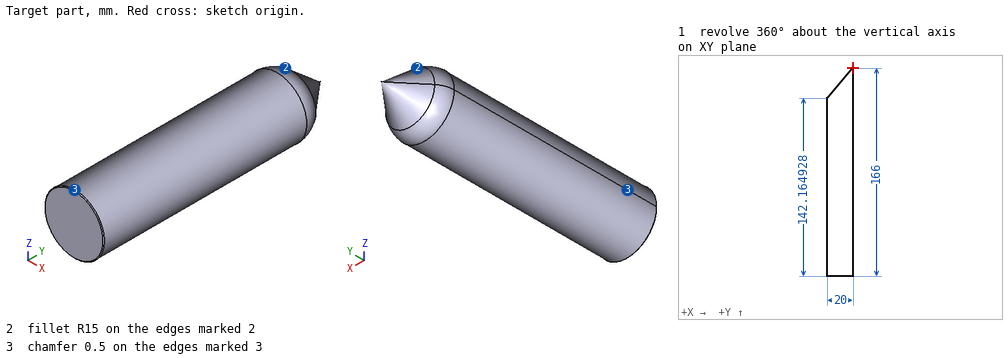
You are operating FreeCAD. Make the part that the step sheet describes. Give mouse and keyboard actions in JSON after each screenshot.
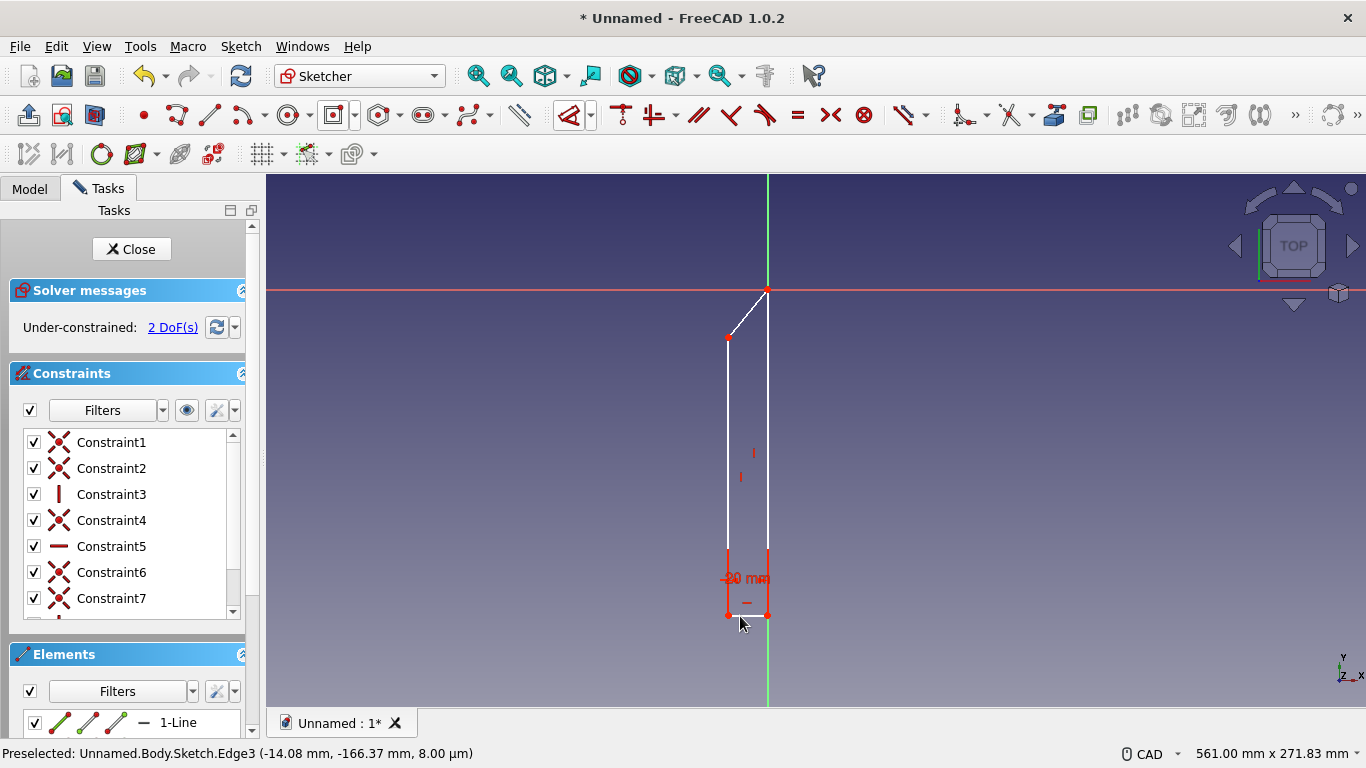
{"action": "left_click", "coordinate": [768, 518]}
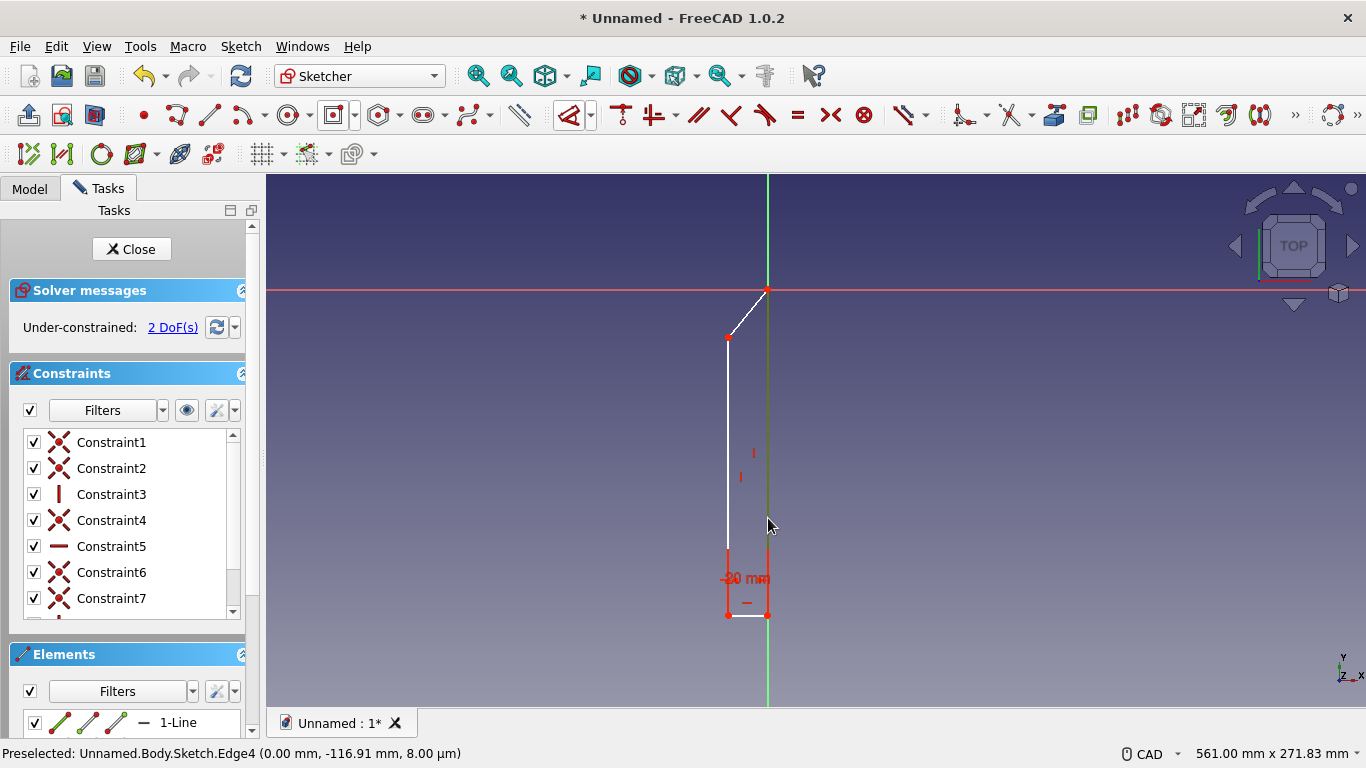
{"action": "left_click", "coordinate": [590, 116]}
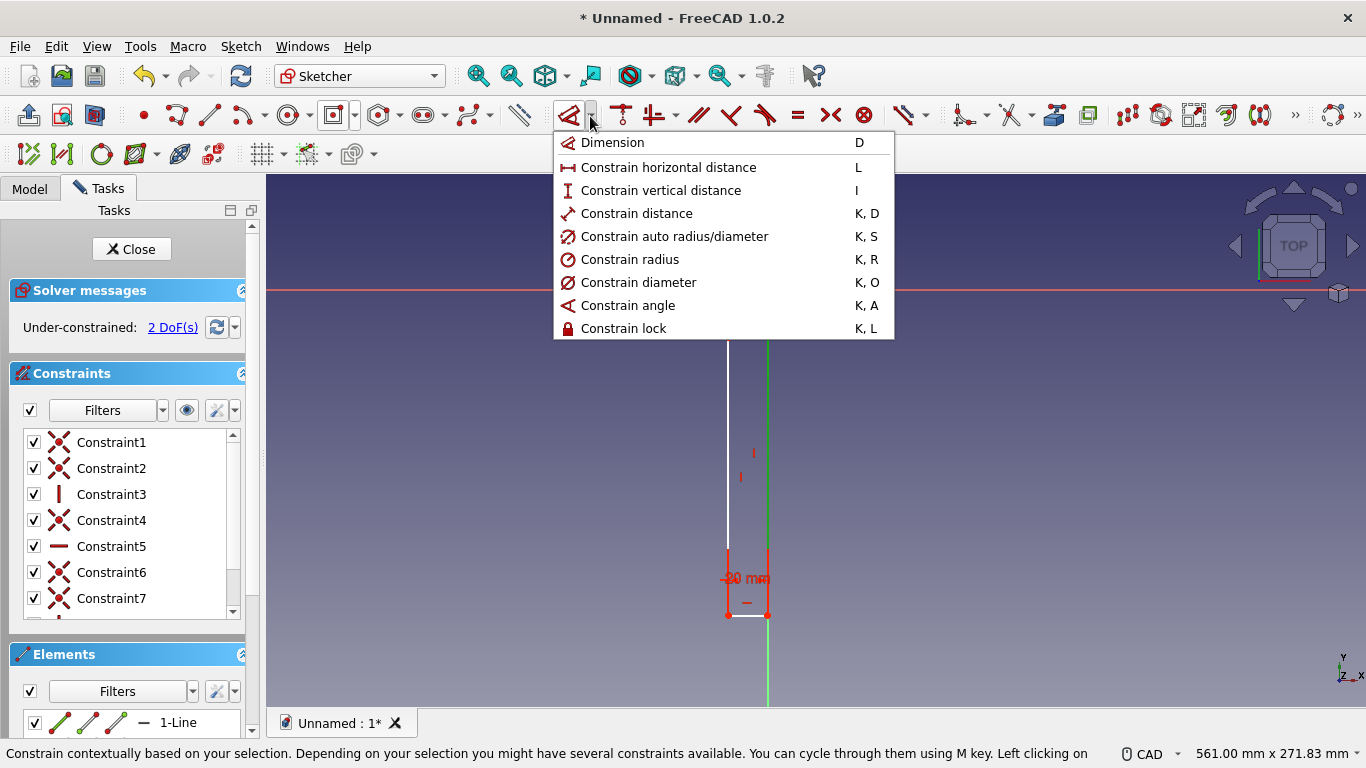
{"action": "left_click", "coordinate": [724, 190]}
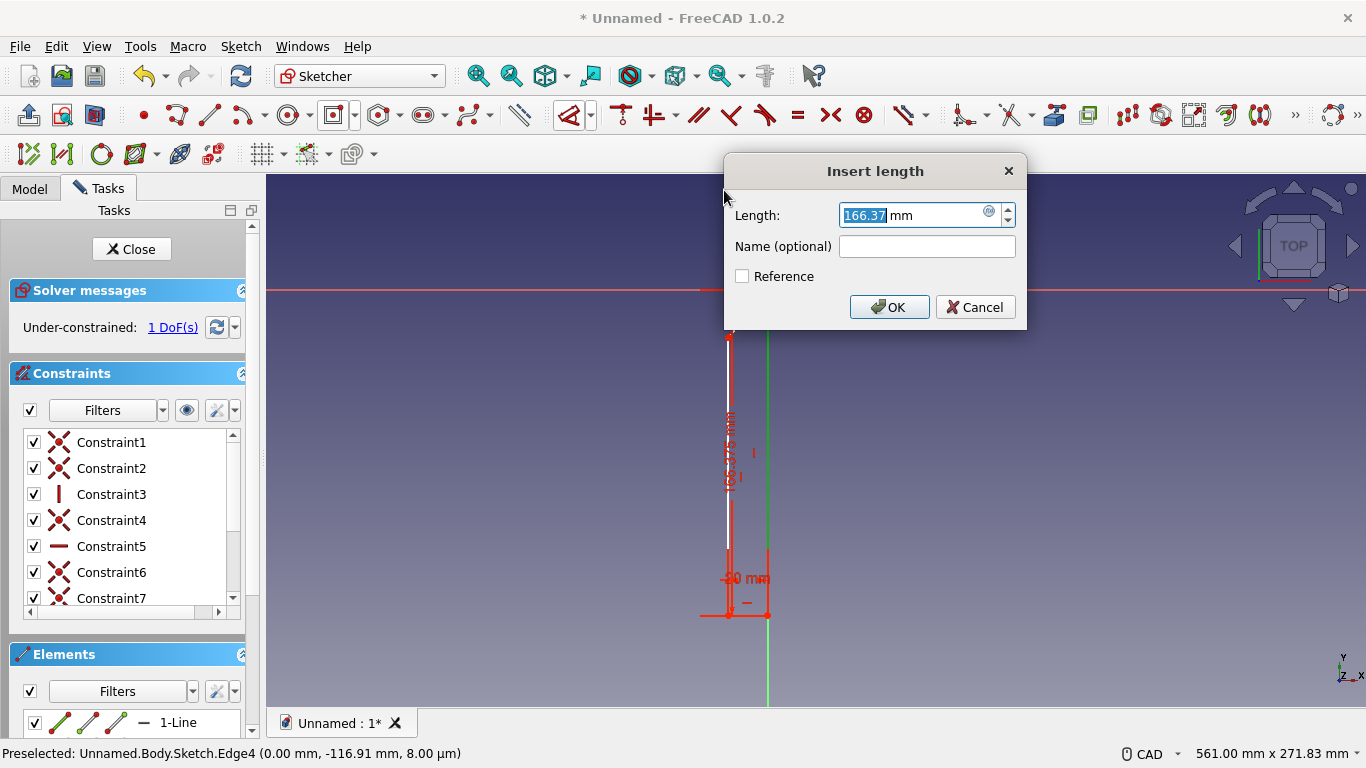
{"action": "type", "text": "166"}
{"action": "key", "text": "Return"}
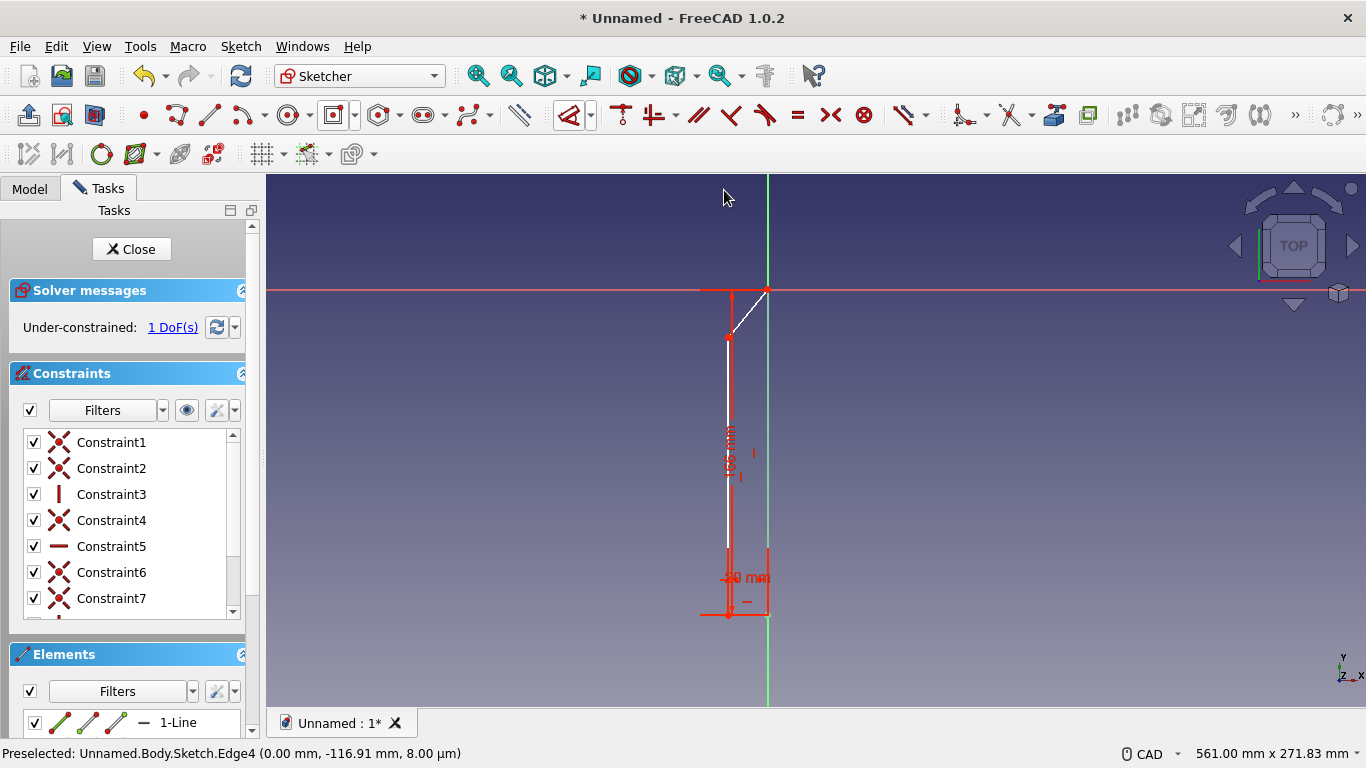
{"action": "left_click", "coordinate": [728, 421]}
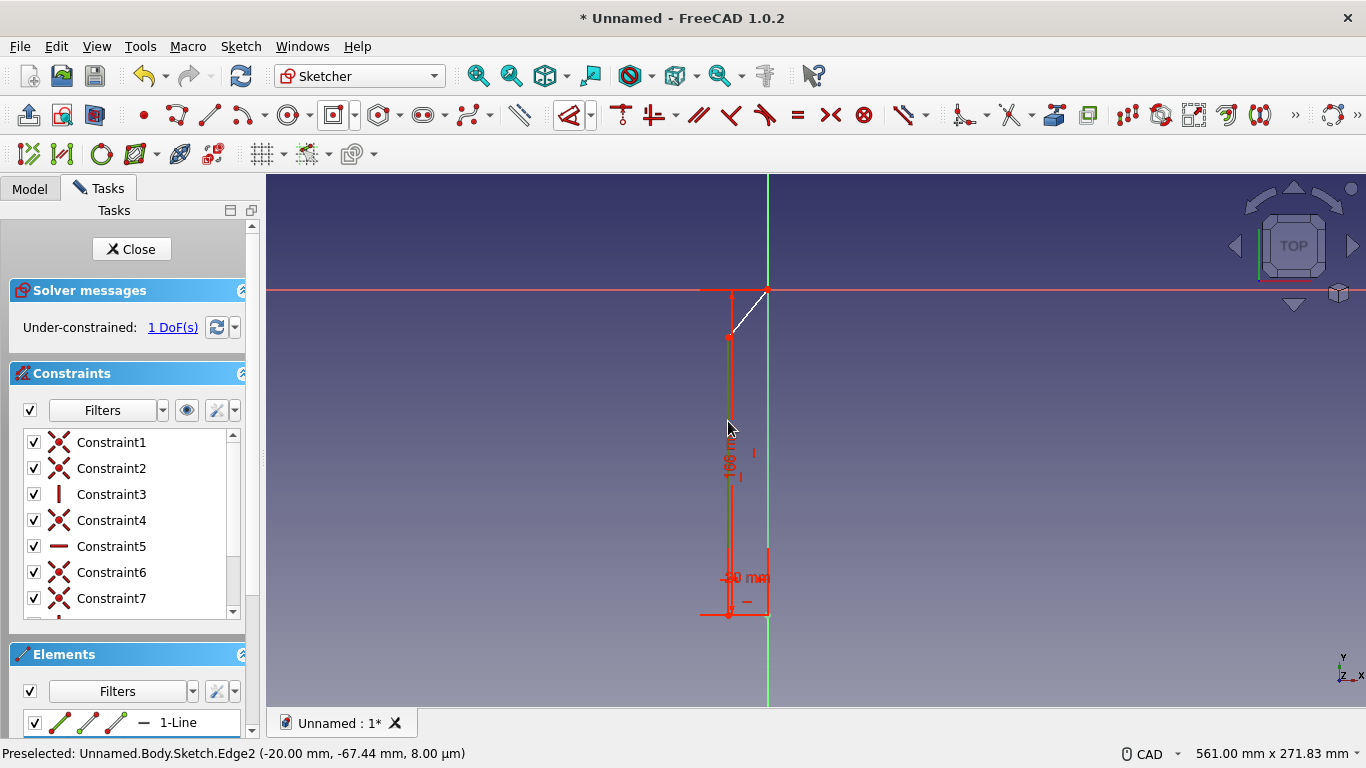
{"action": "left_click", "coordinate": [590, 116]}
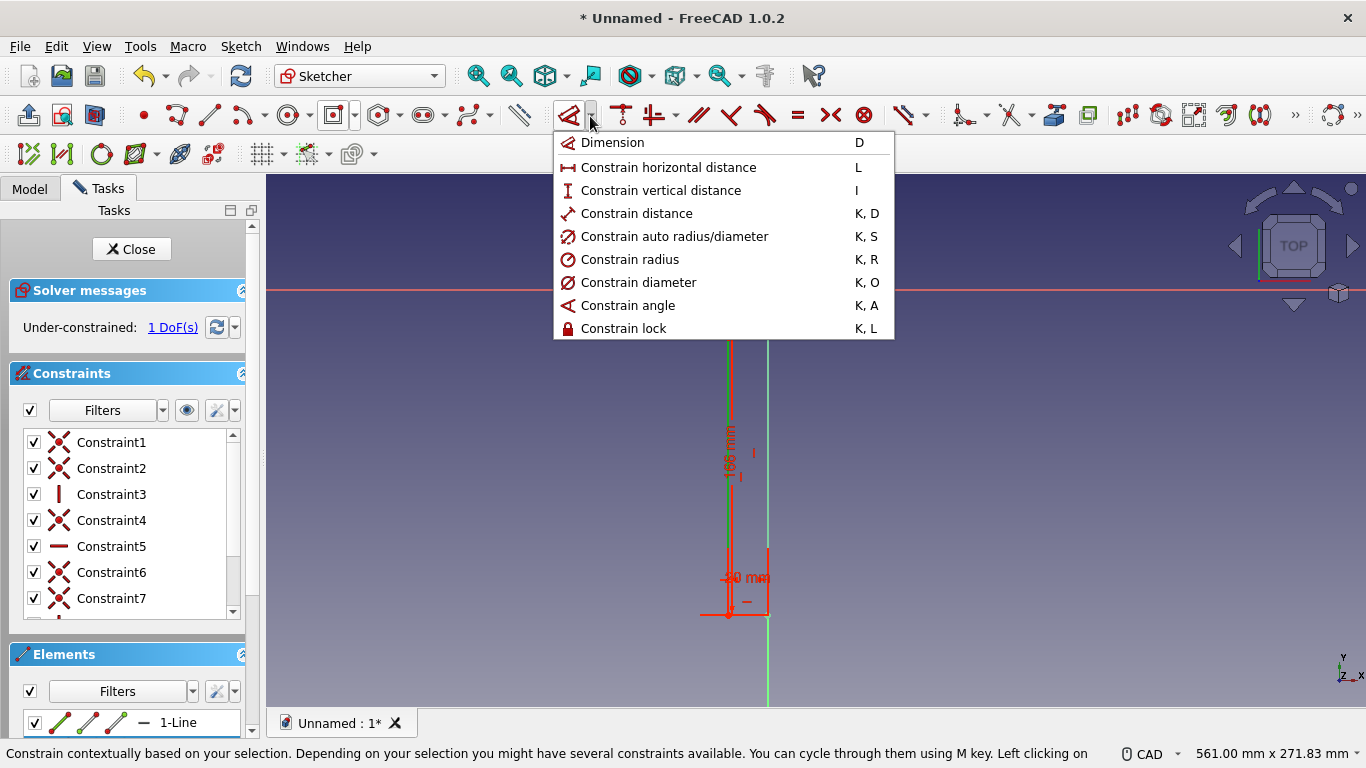
{"action": "left_click", "coordinate": [724, 190]}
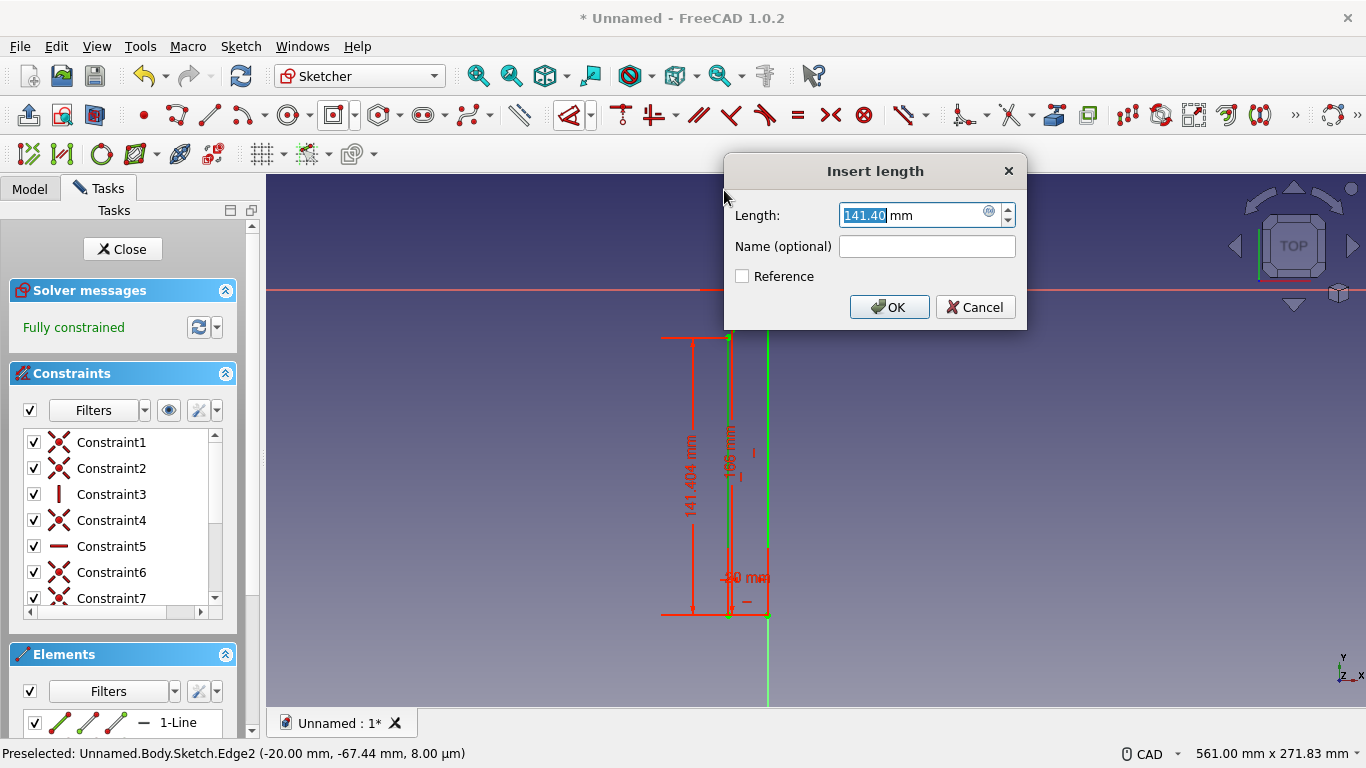
{"action": "type", "text": "142.164928"}
{"action": "key", "text": "Return"}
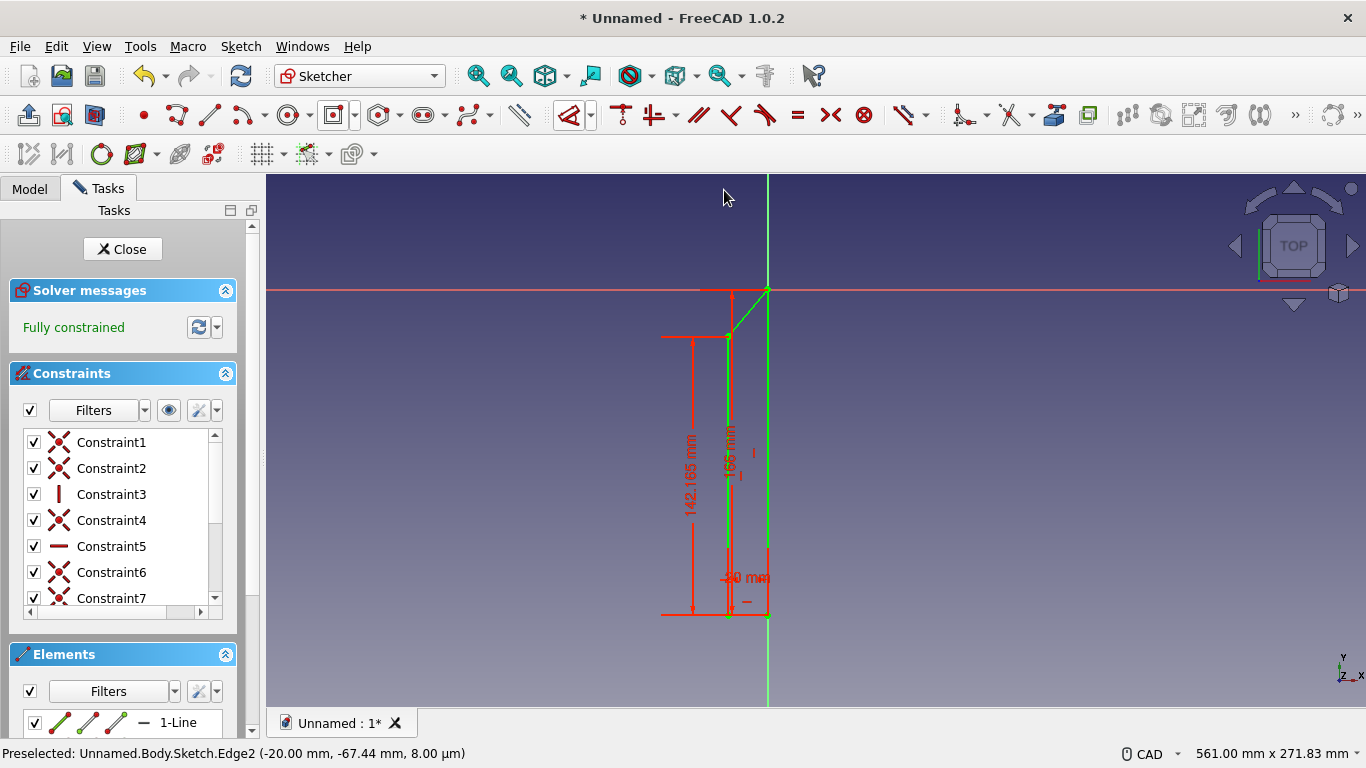
{"action": "left_click", "coordinate": [123, 249]}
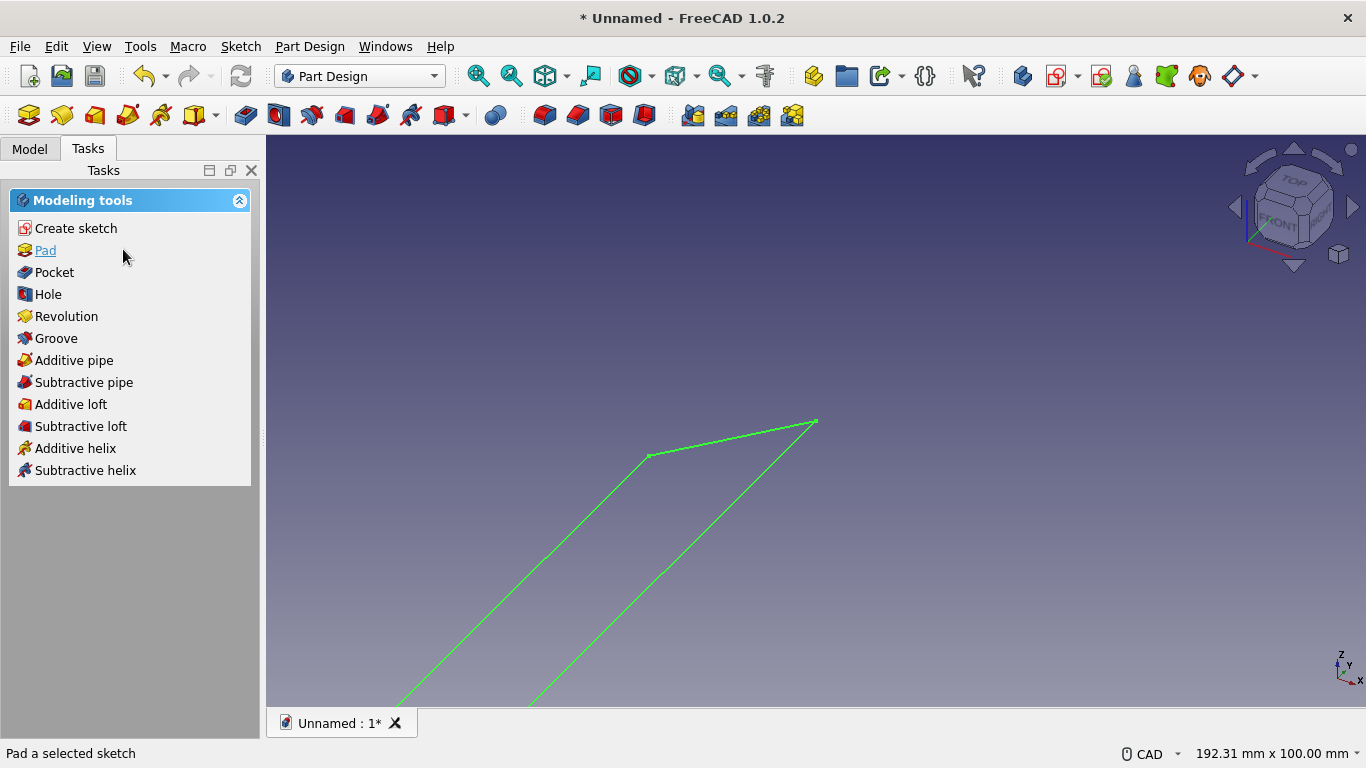
{"action": "left_click", "coordinate": [62, 116]}